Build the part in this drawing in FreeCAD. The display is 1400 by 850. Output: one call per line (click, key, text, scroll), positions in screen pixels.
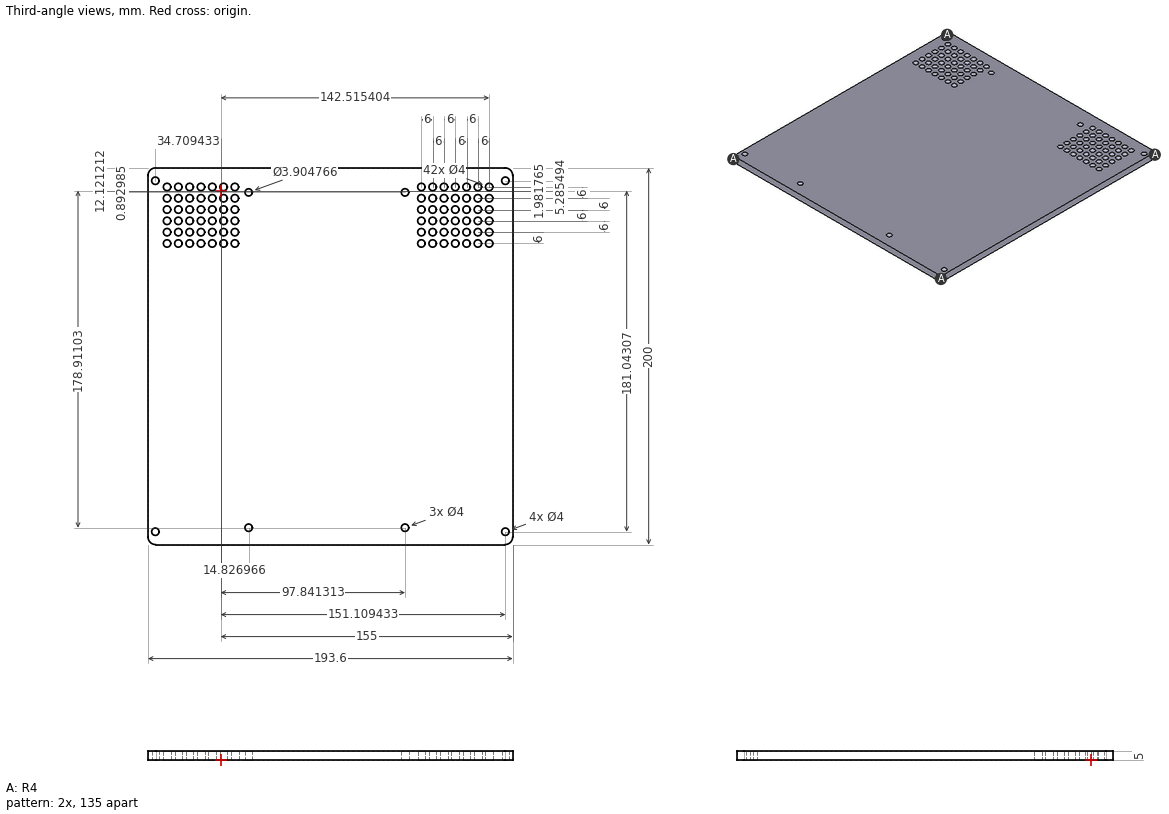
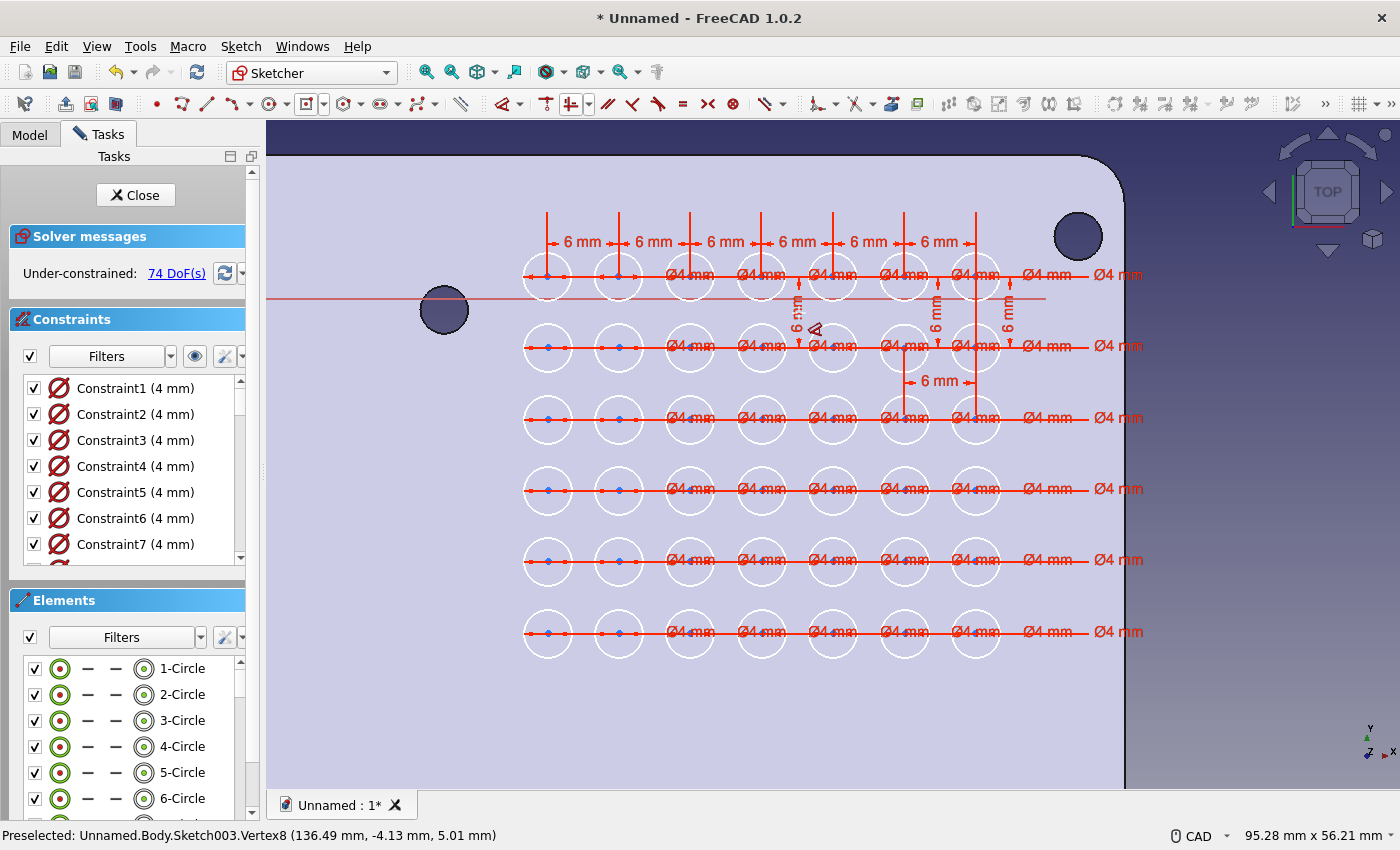
click(761, 277)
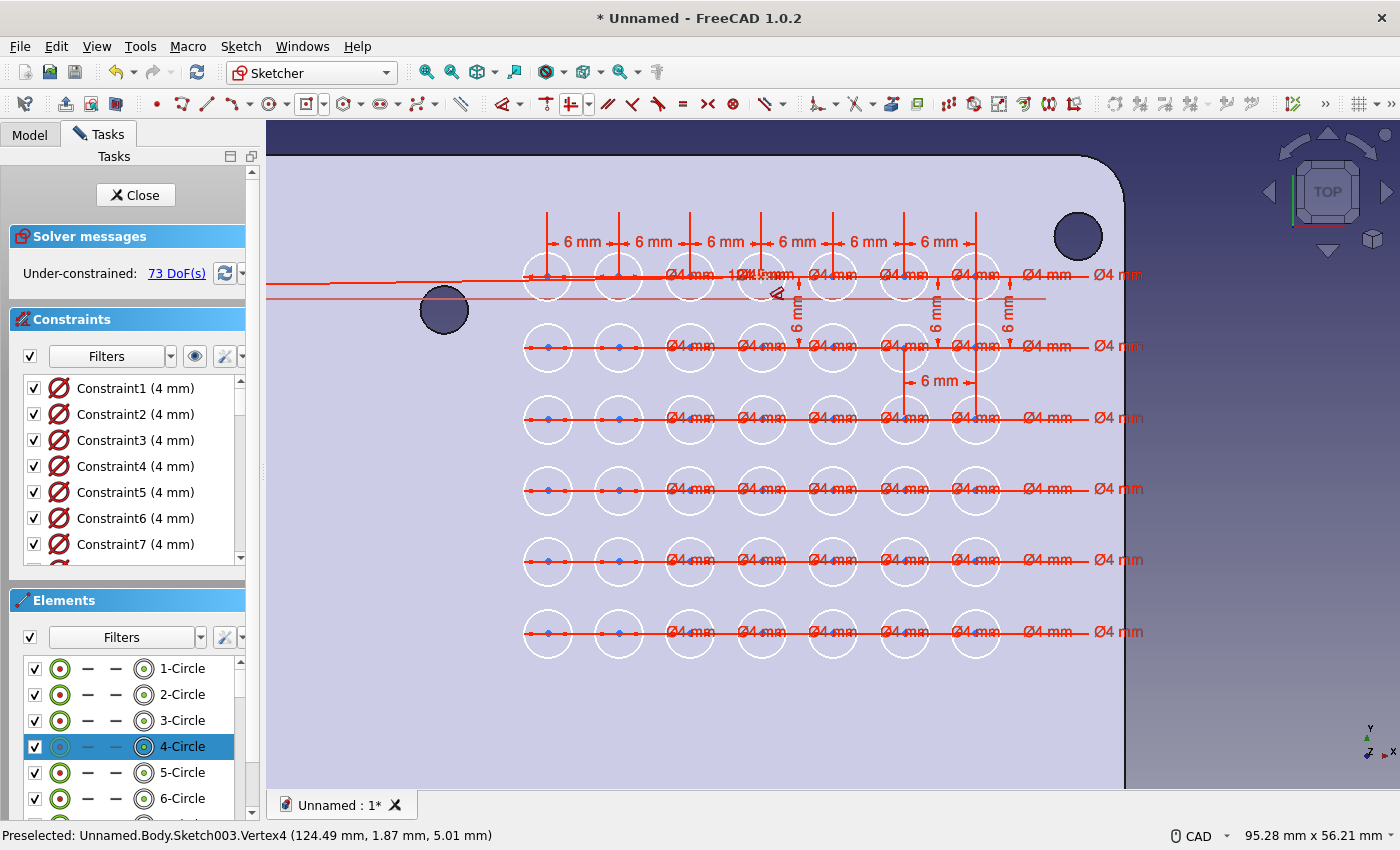
click(904, 348)
click(727, 313)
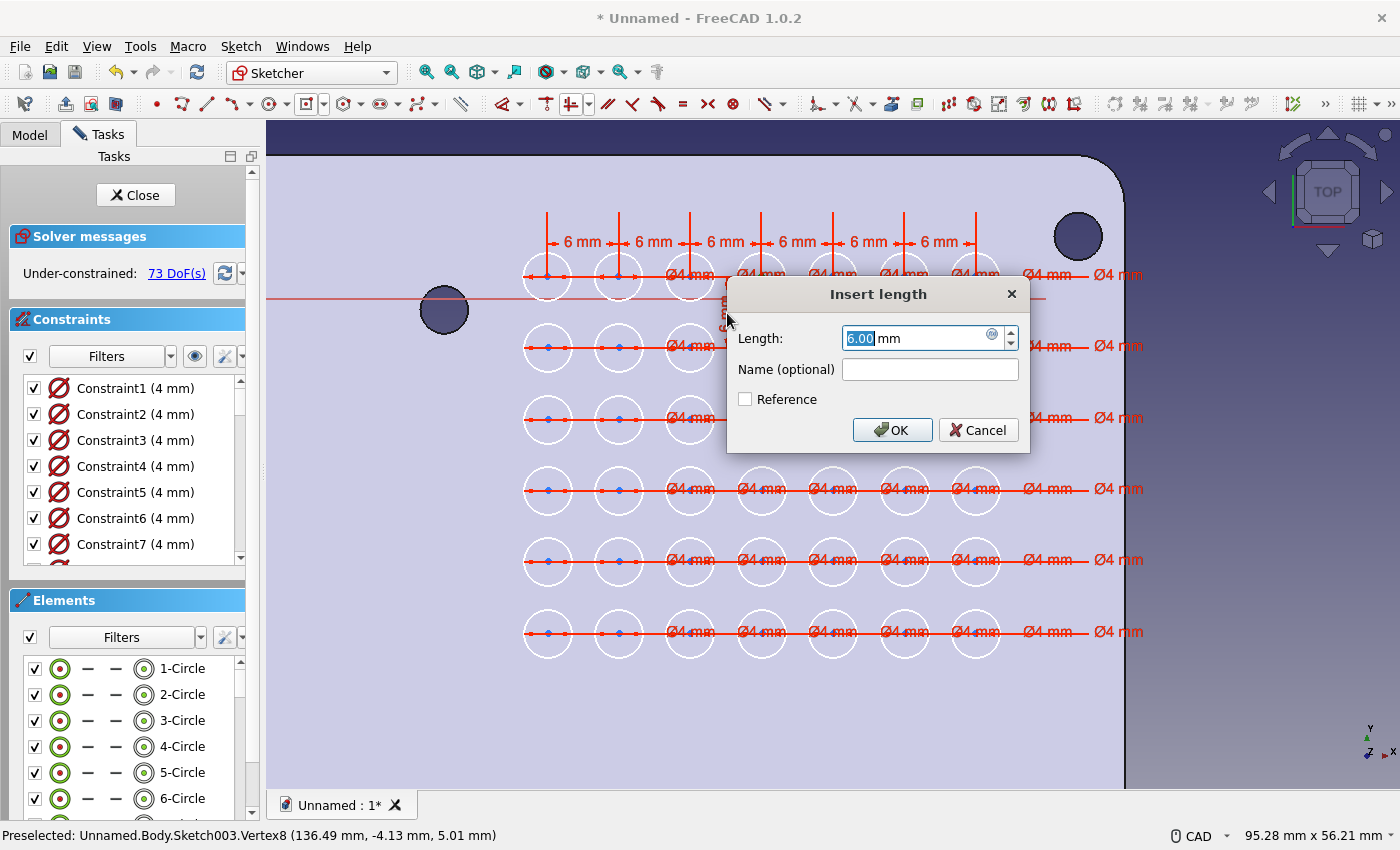
text(6)
key(Return)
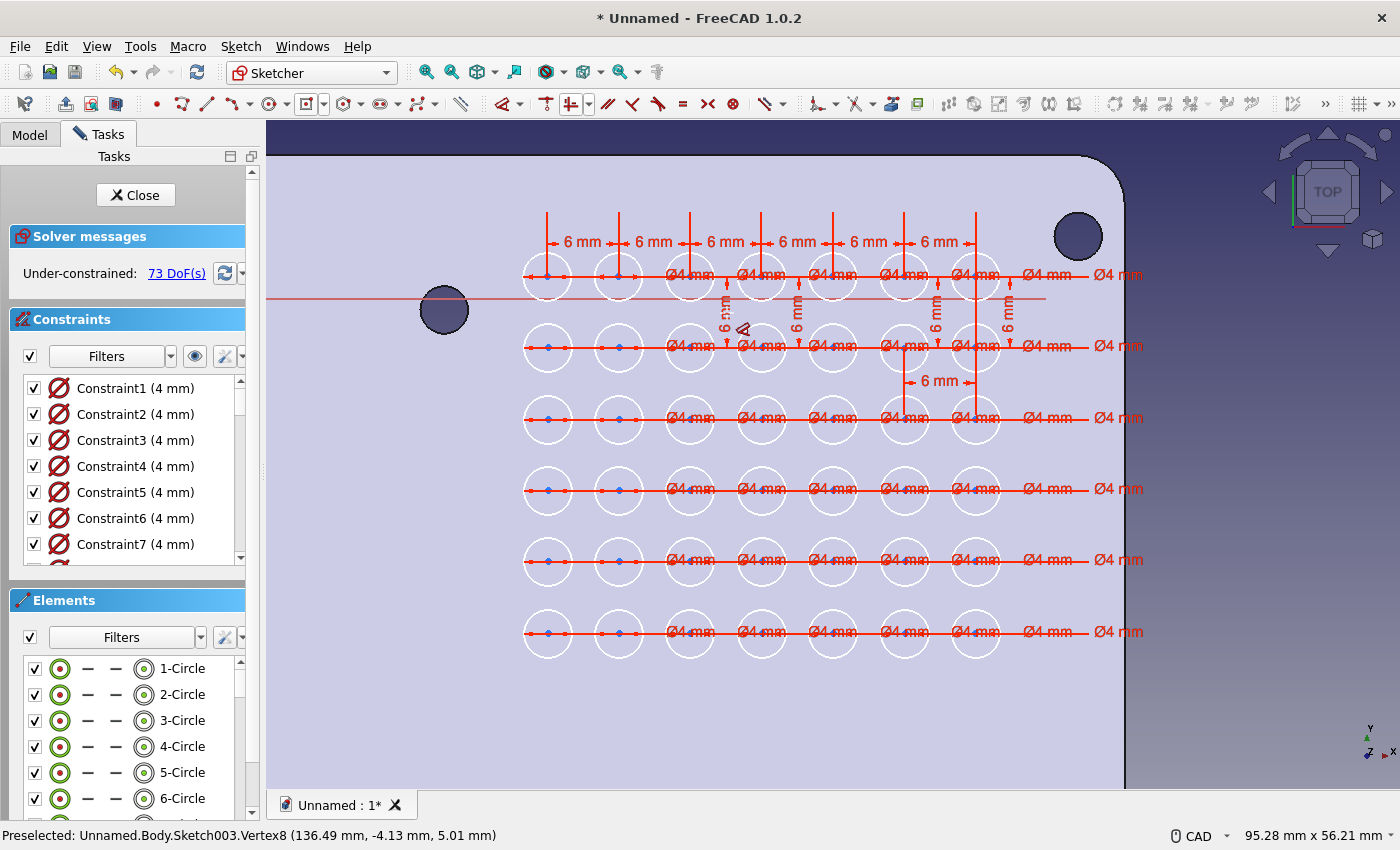
click(690, 277)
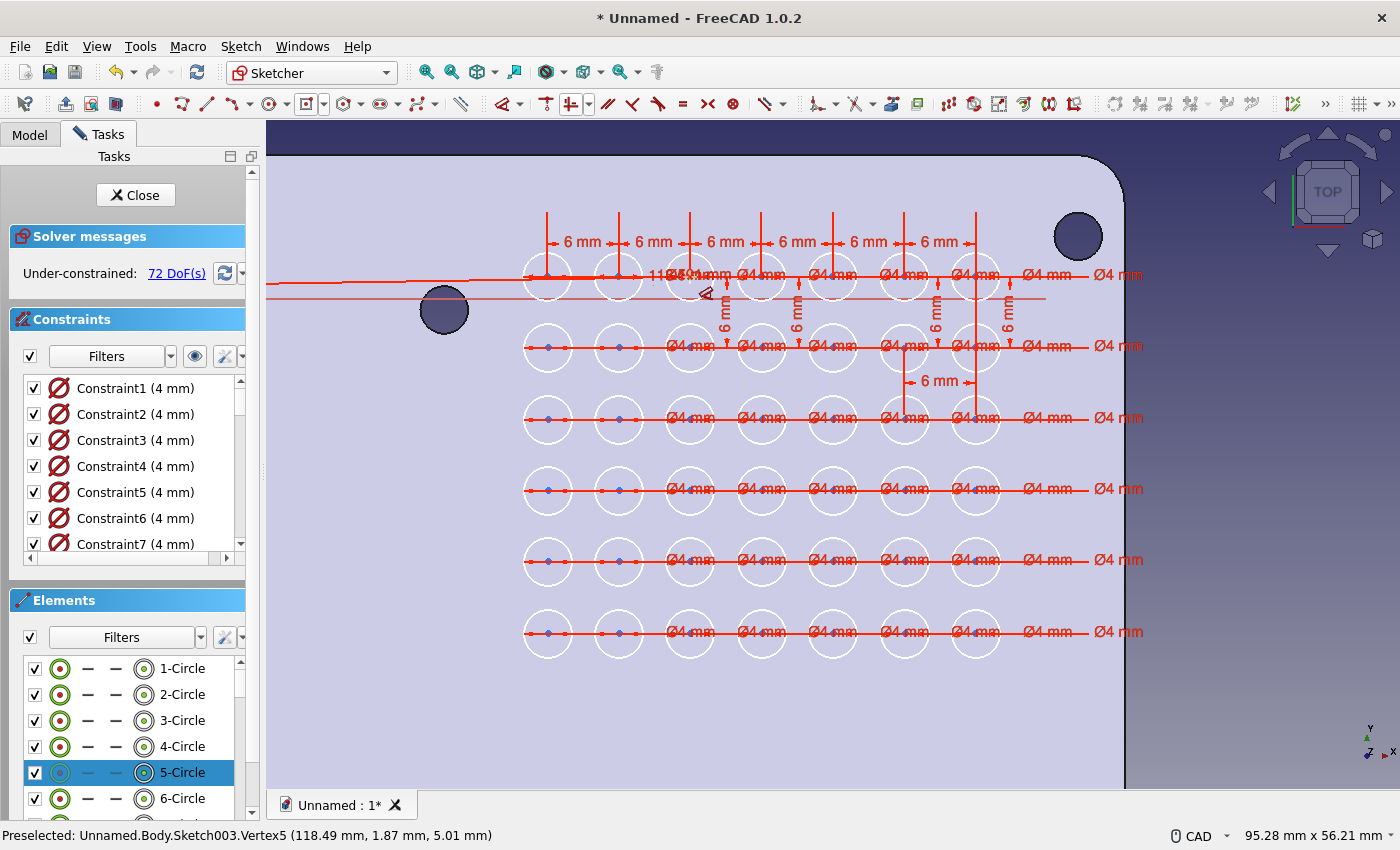
click(904, 348)
click(656, 313)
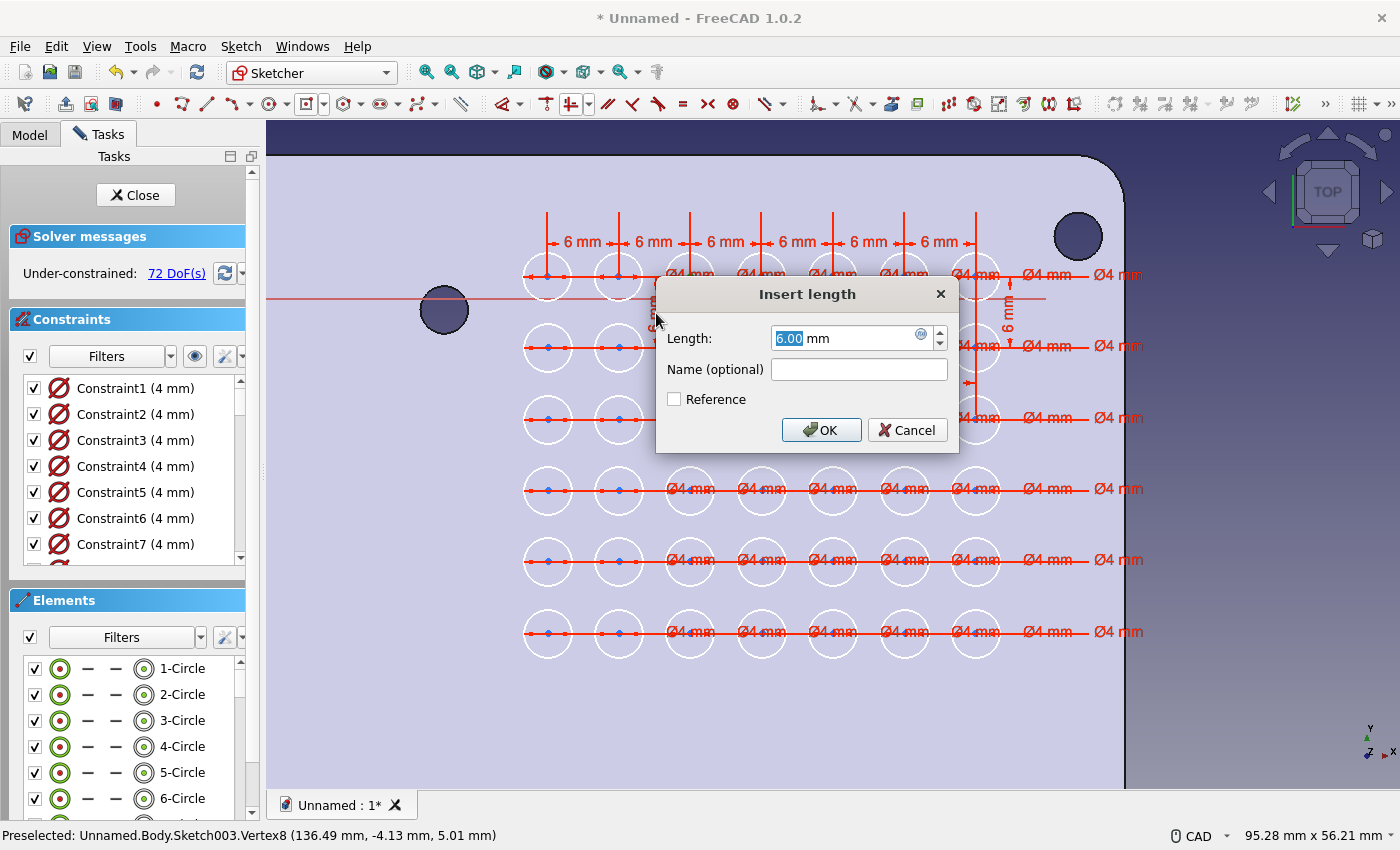
text(6)
key(Return)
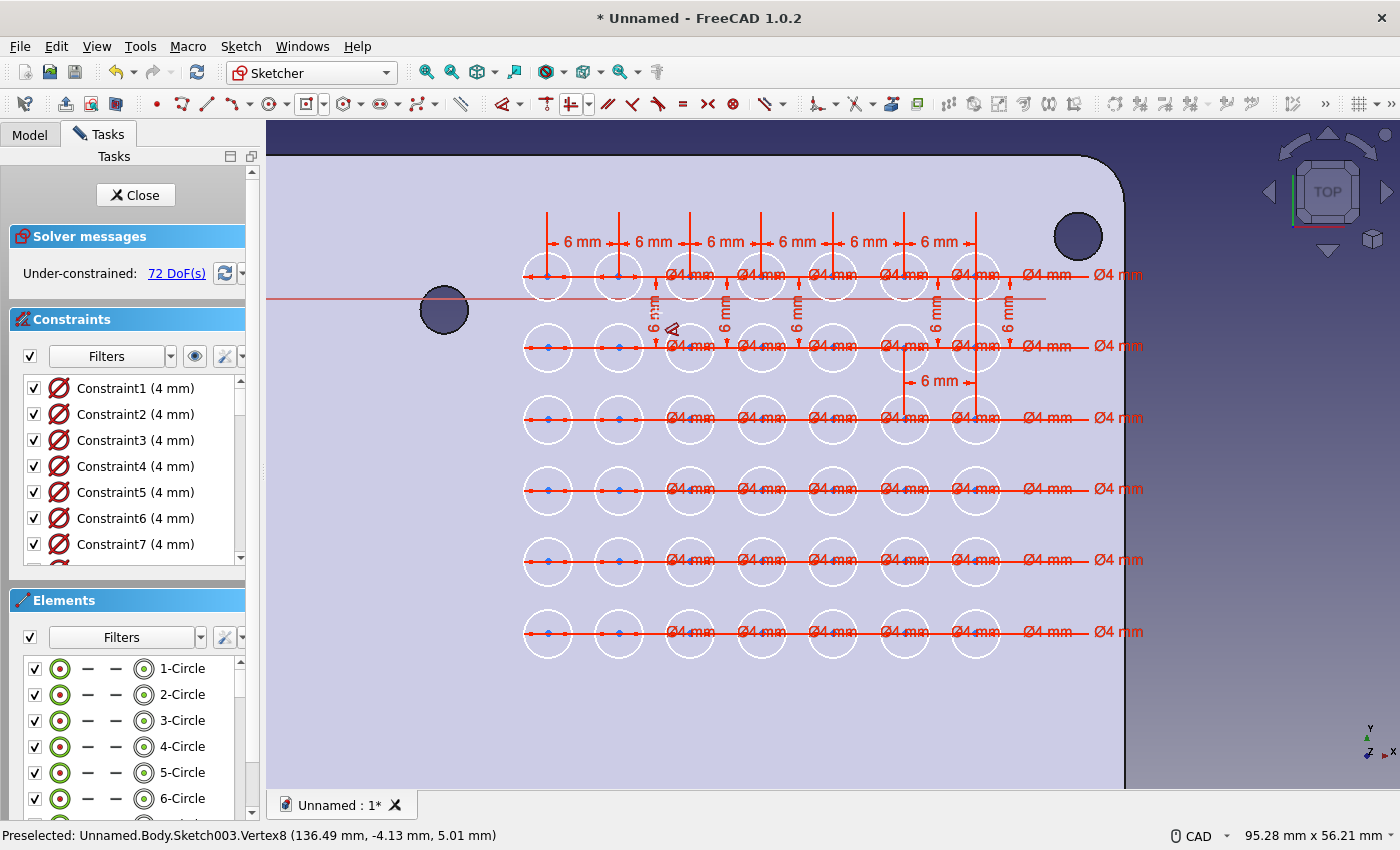
click(619, 277)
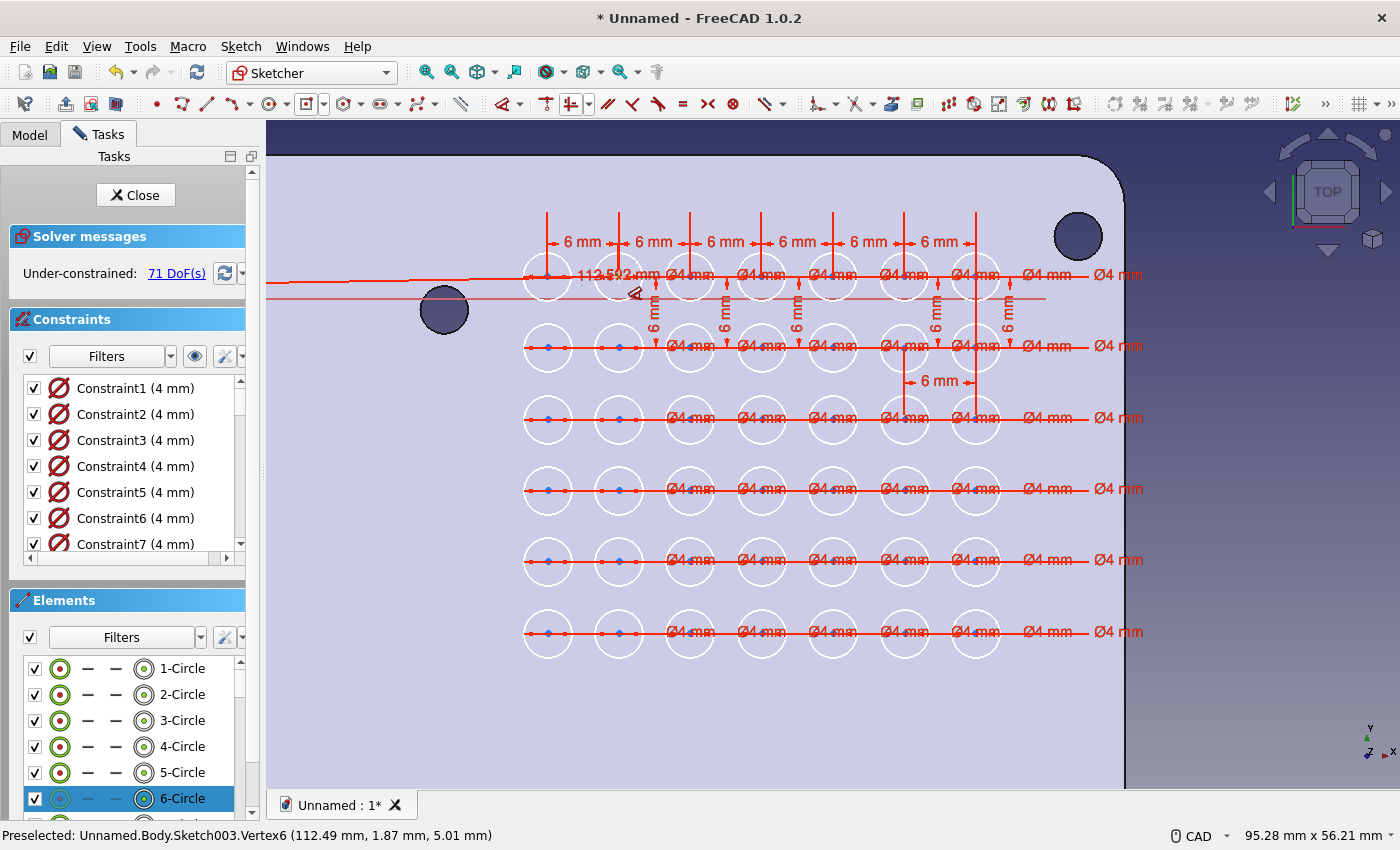
click(904, 348)
click(585, 313)